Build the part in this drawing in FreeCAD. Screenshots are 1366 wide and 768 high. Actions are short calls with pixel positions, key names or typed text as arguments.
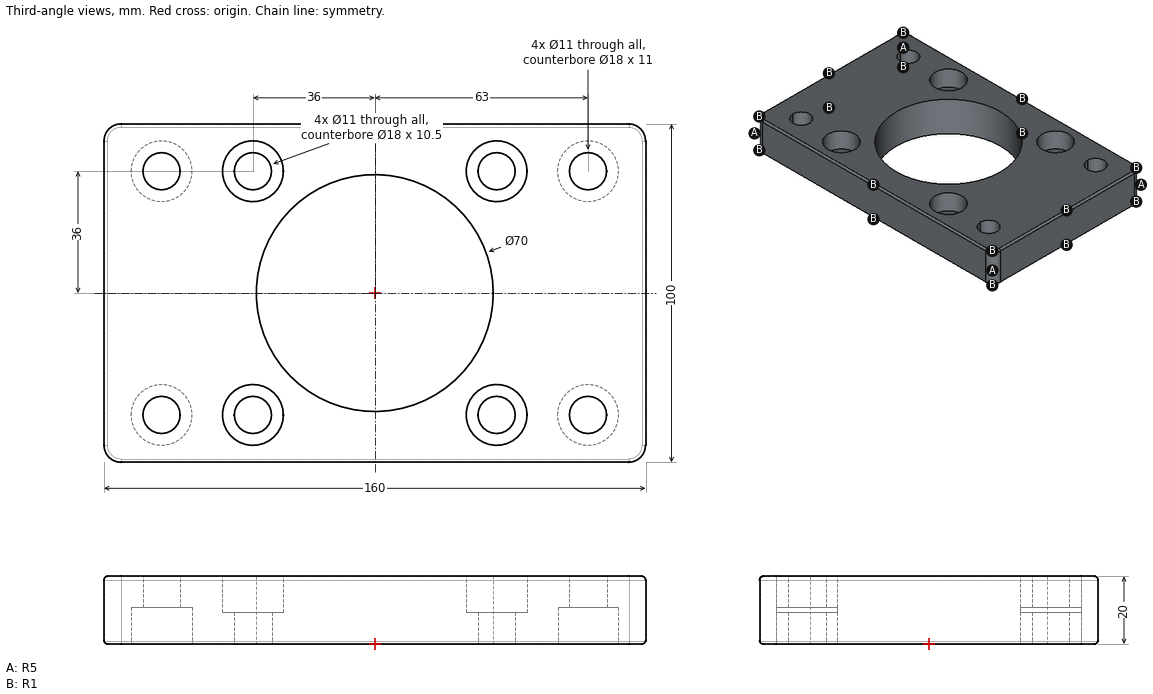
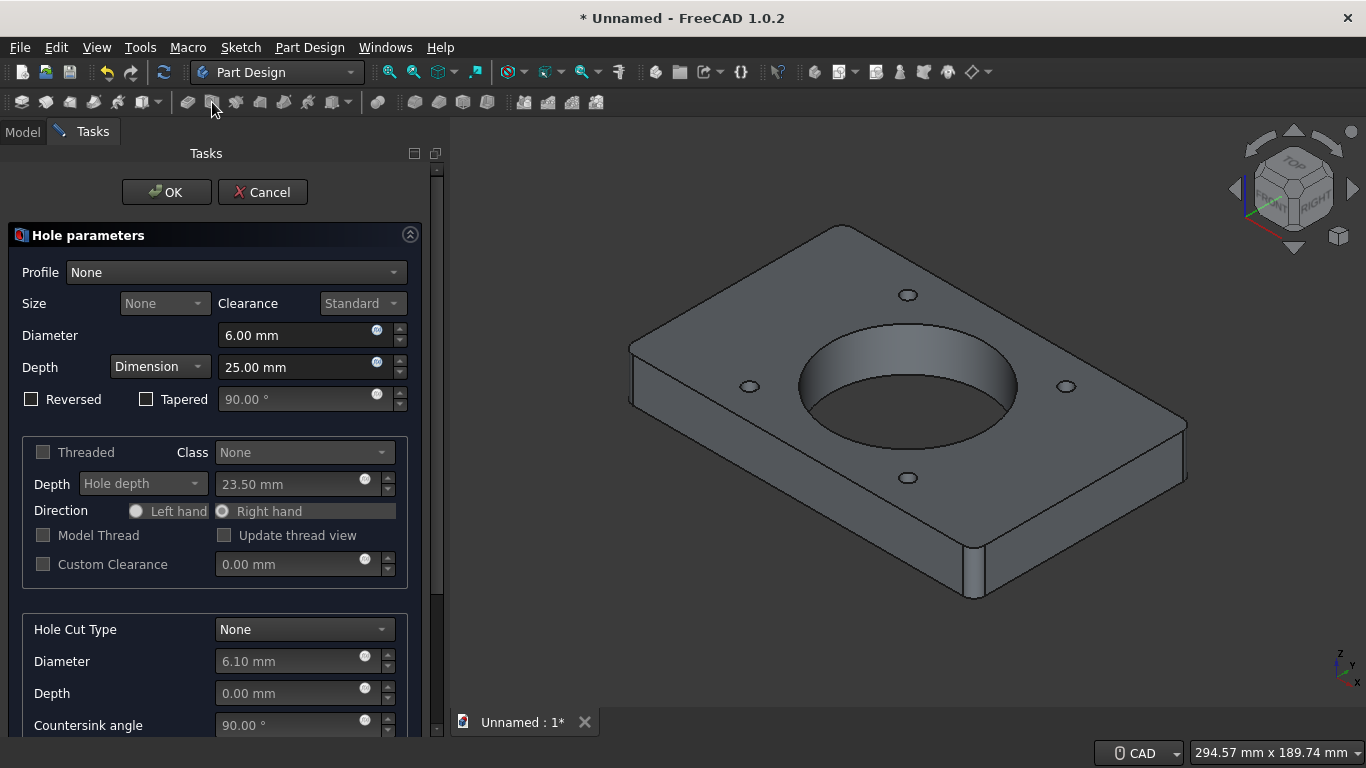
triple_click(305, 335)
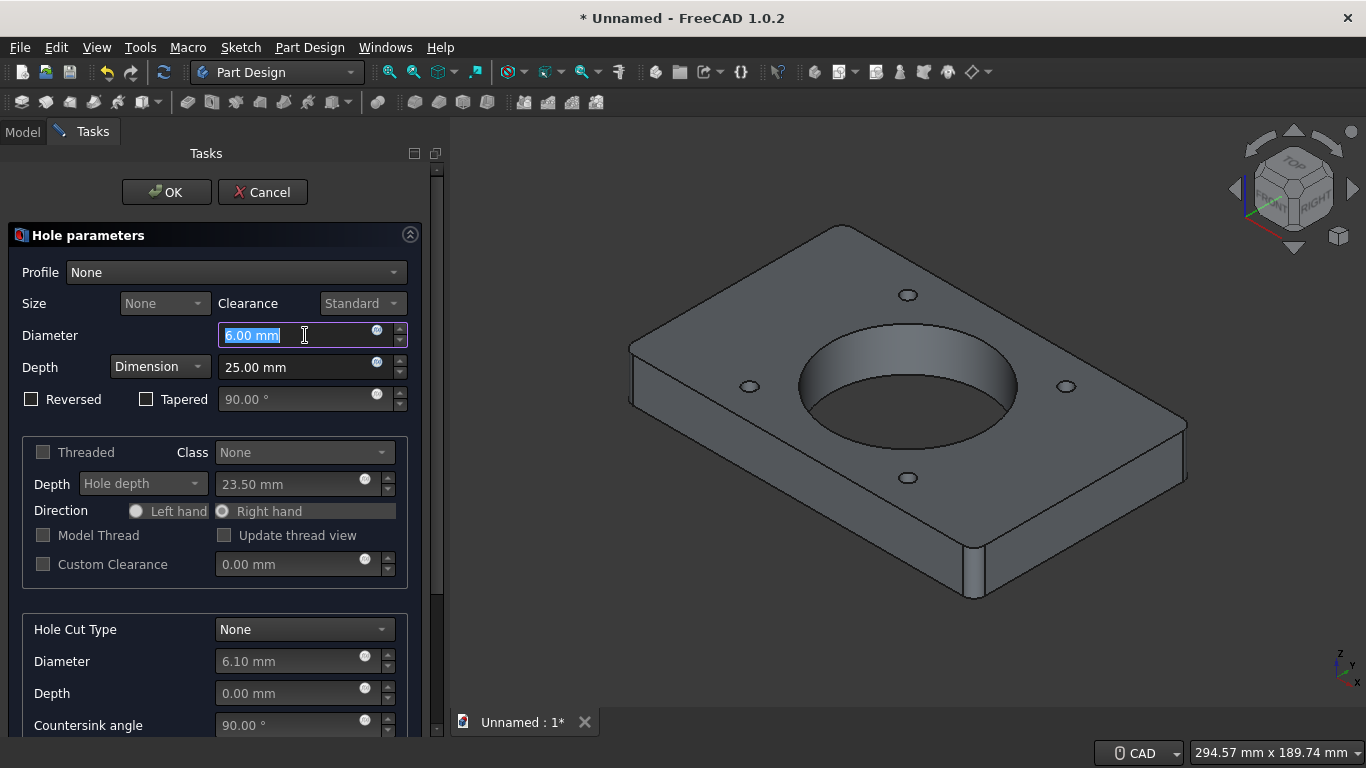
text(11)
key(Tab)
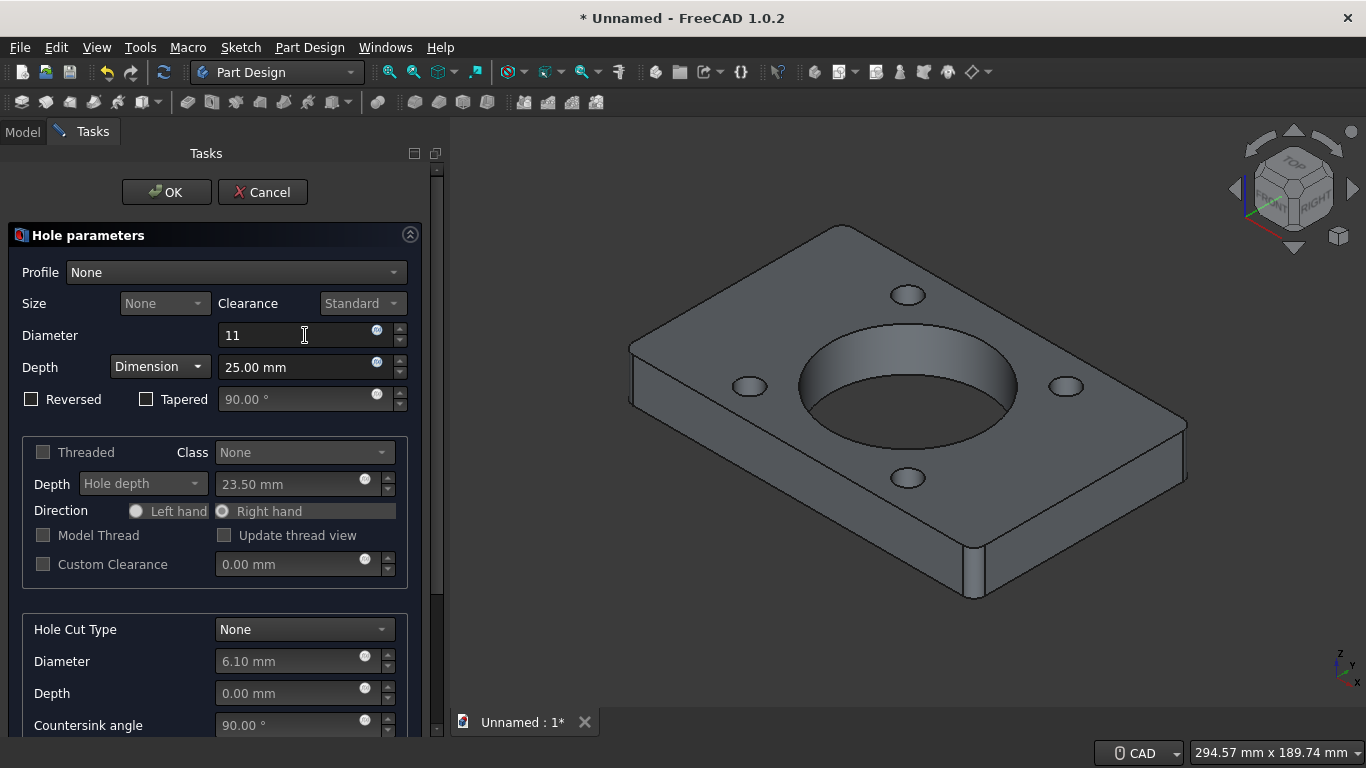
click(161, 366)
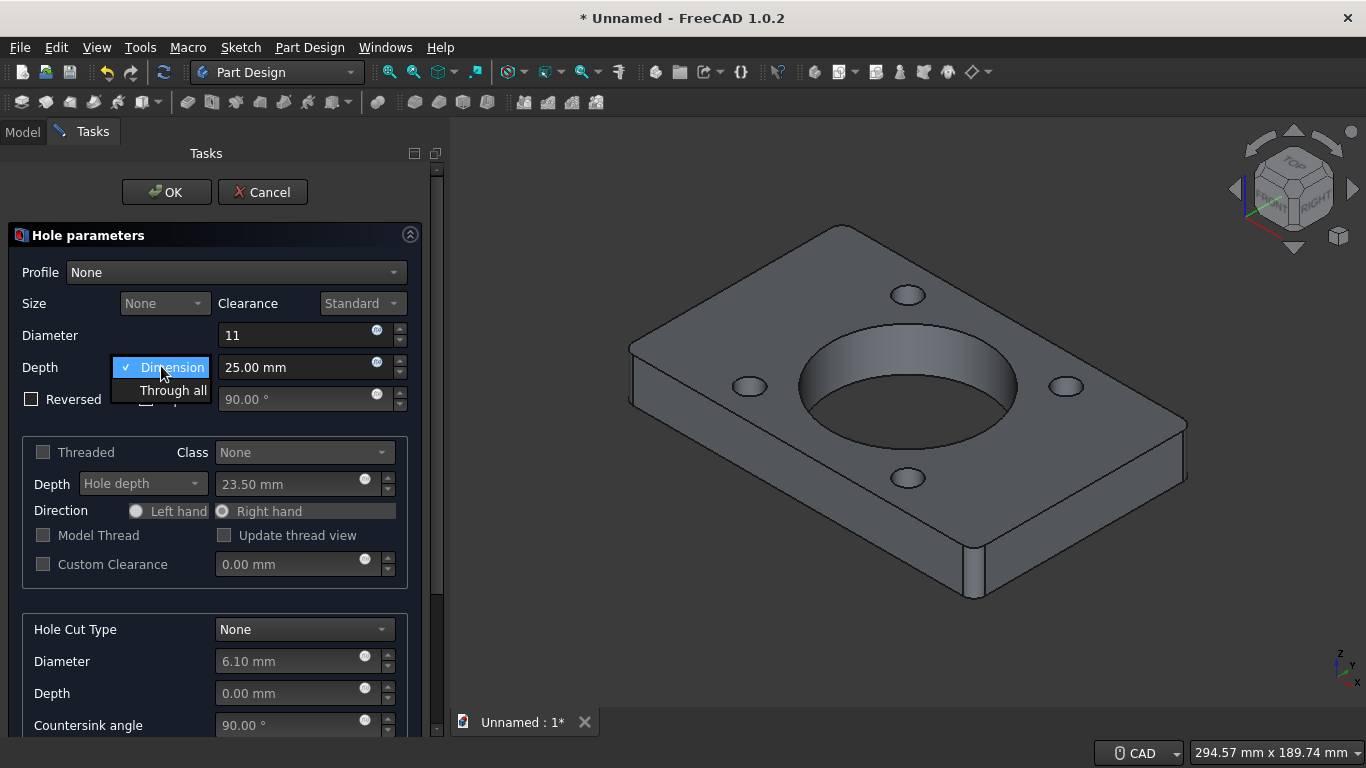
click(160, 390)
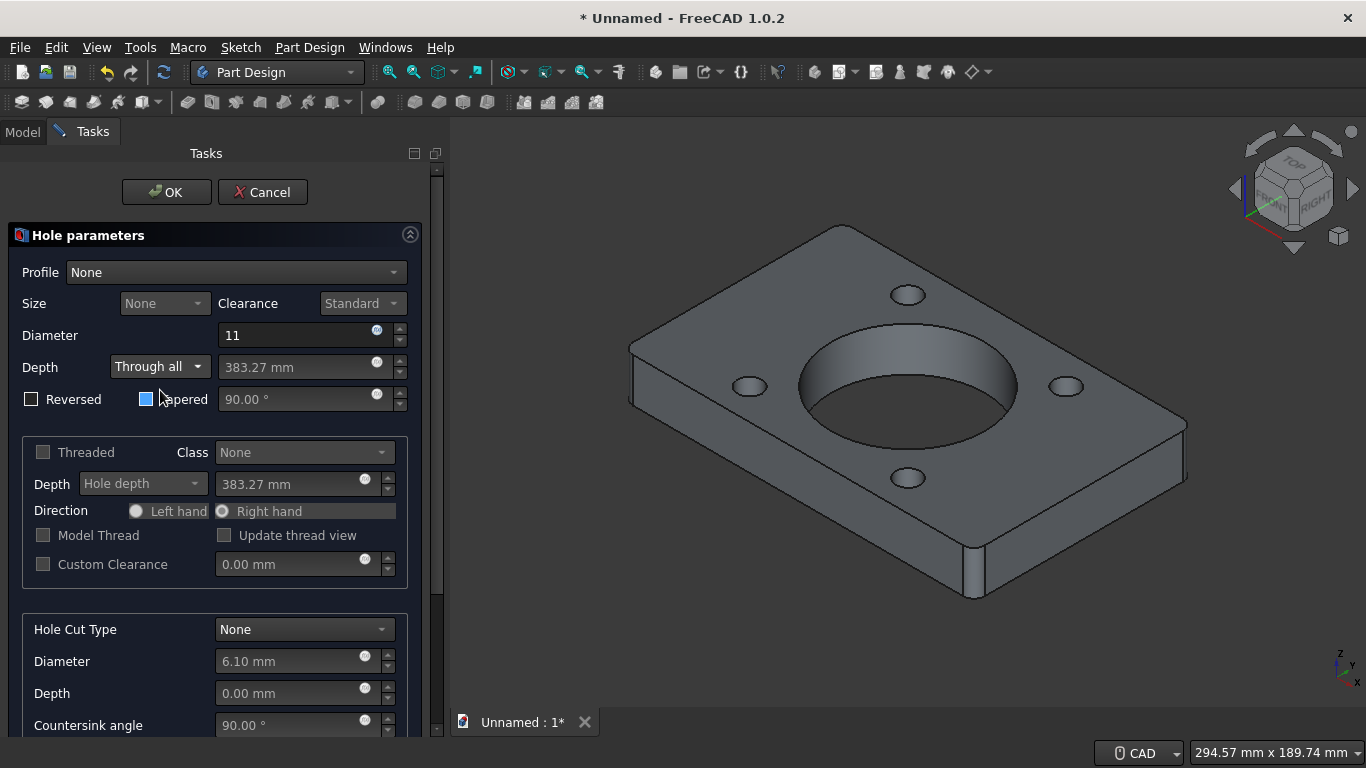
click(306, 630)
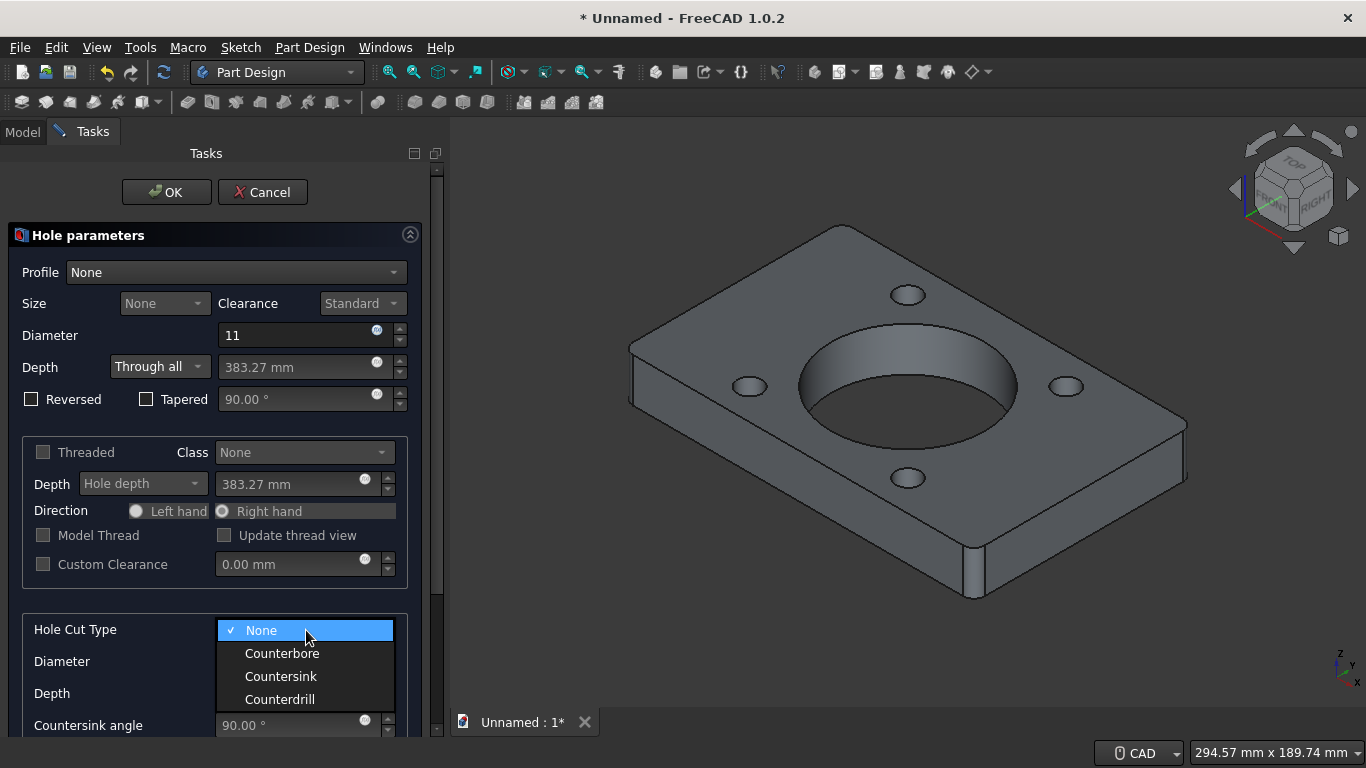
click(304, 654)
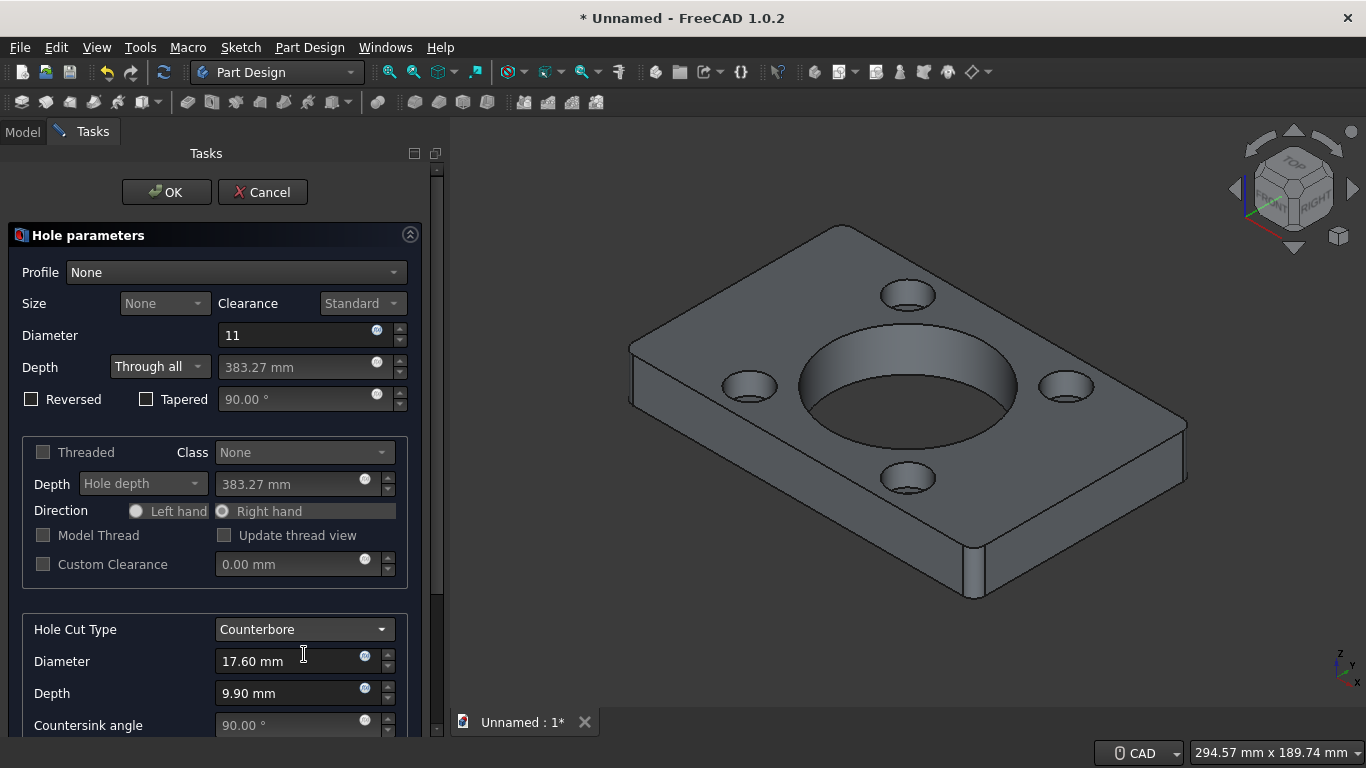
triple_click(298, 661)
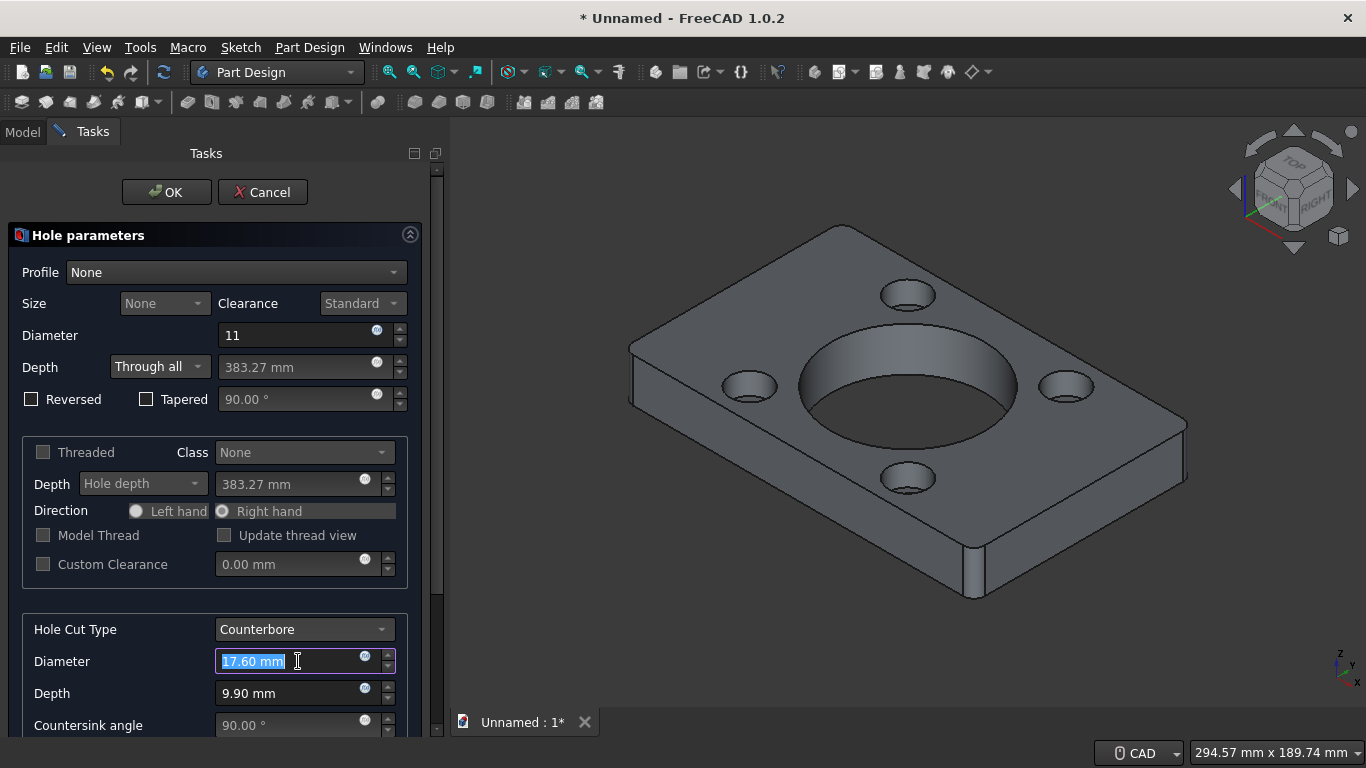
text(18)
key(Tab)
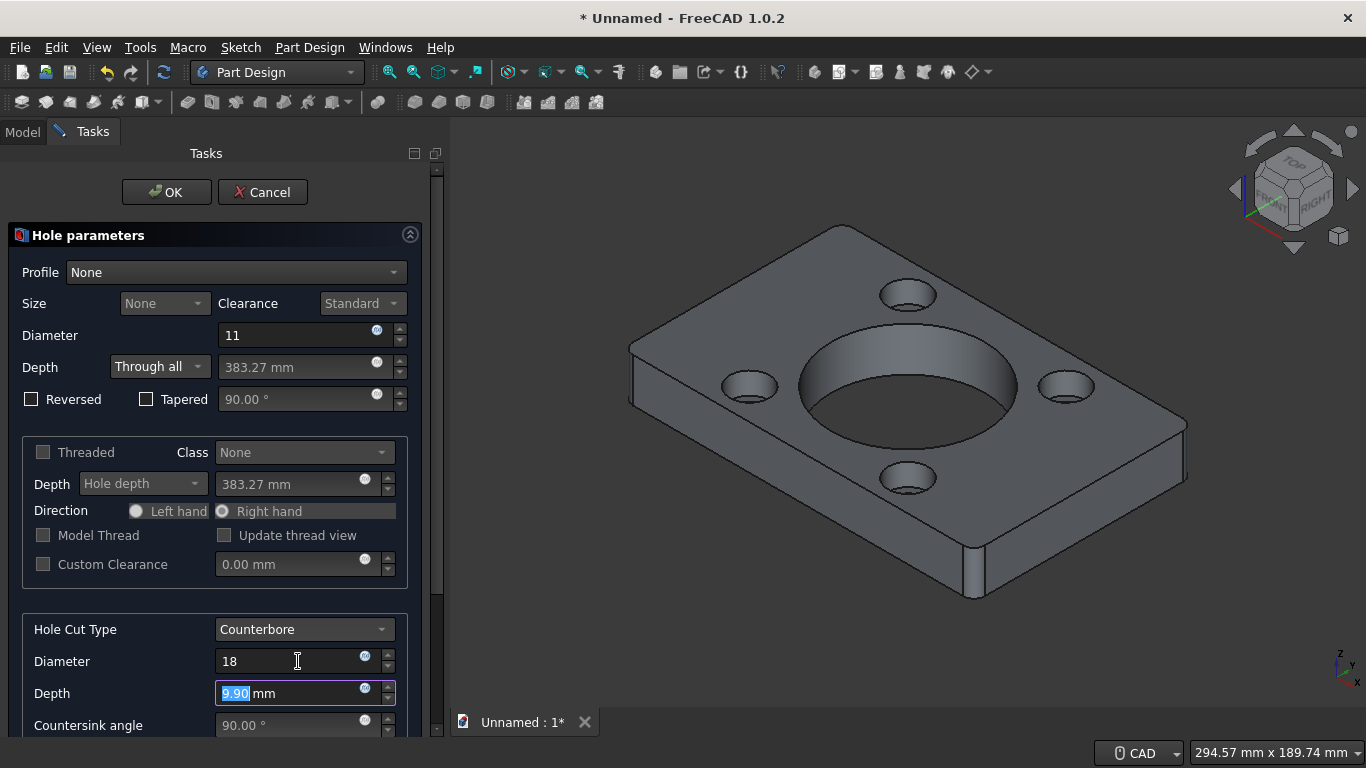
text(10.5)
key(Tab)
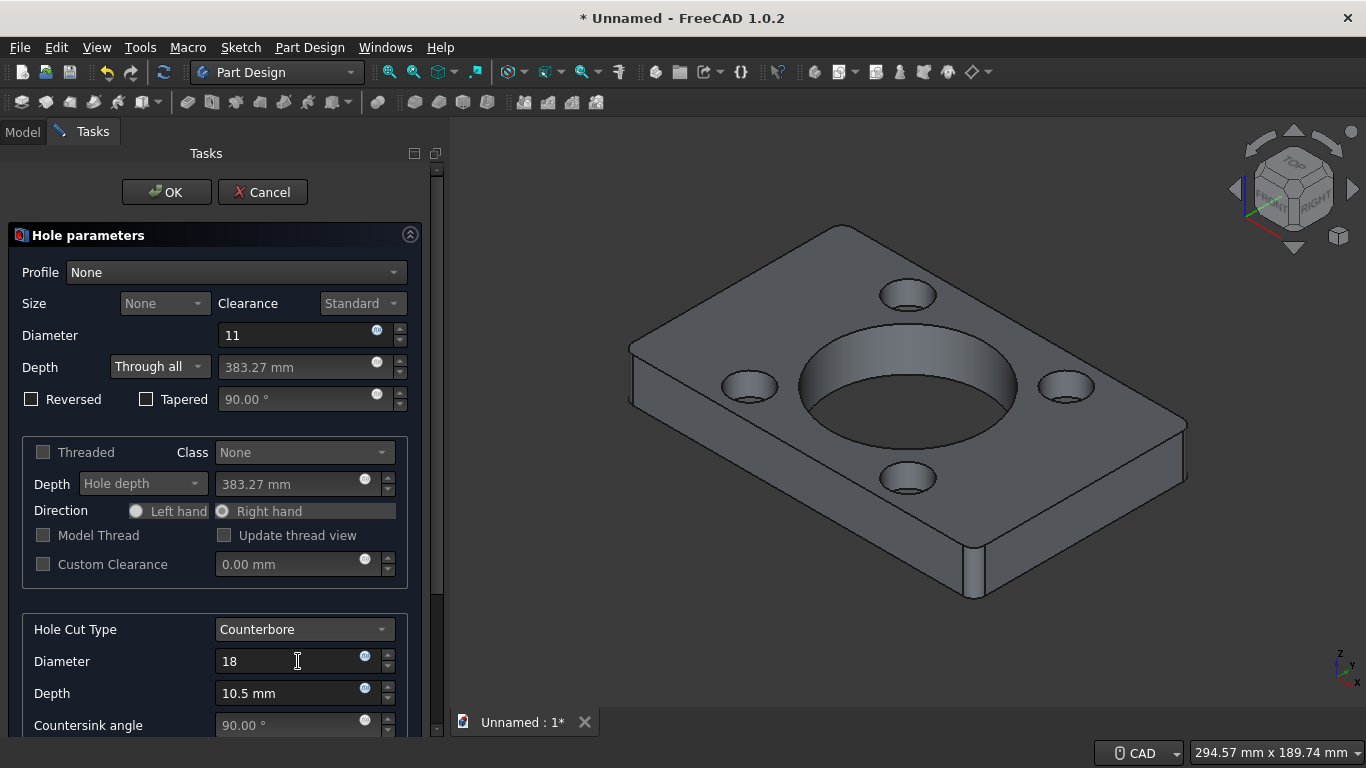
click(167, 192)